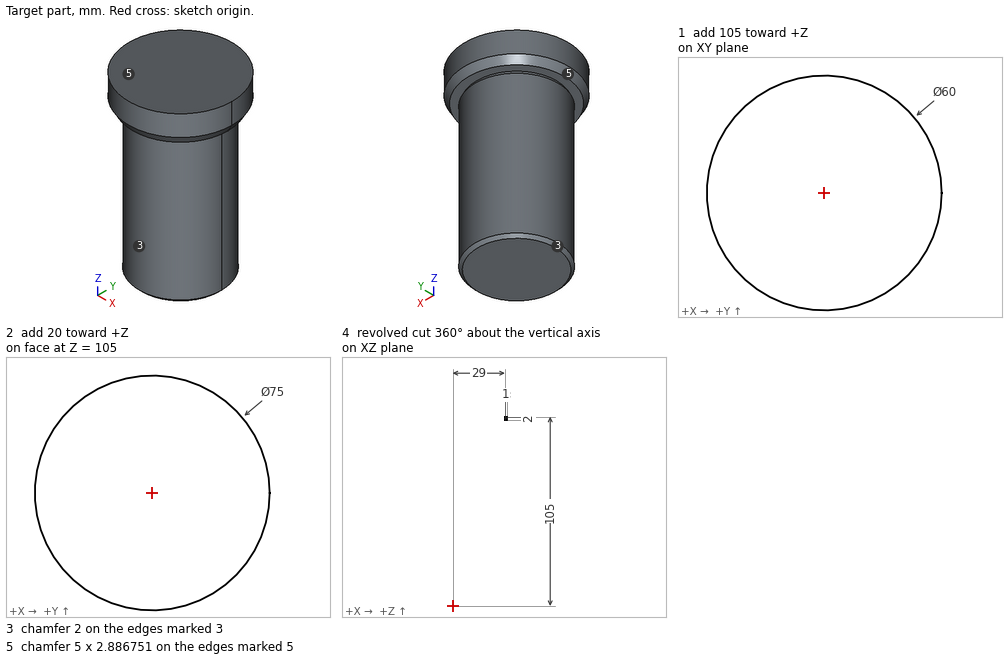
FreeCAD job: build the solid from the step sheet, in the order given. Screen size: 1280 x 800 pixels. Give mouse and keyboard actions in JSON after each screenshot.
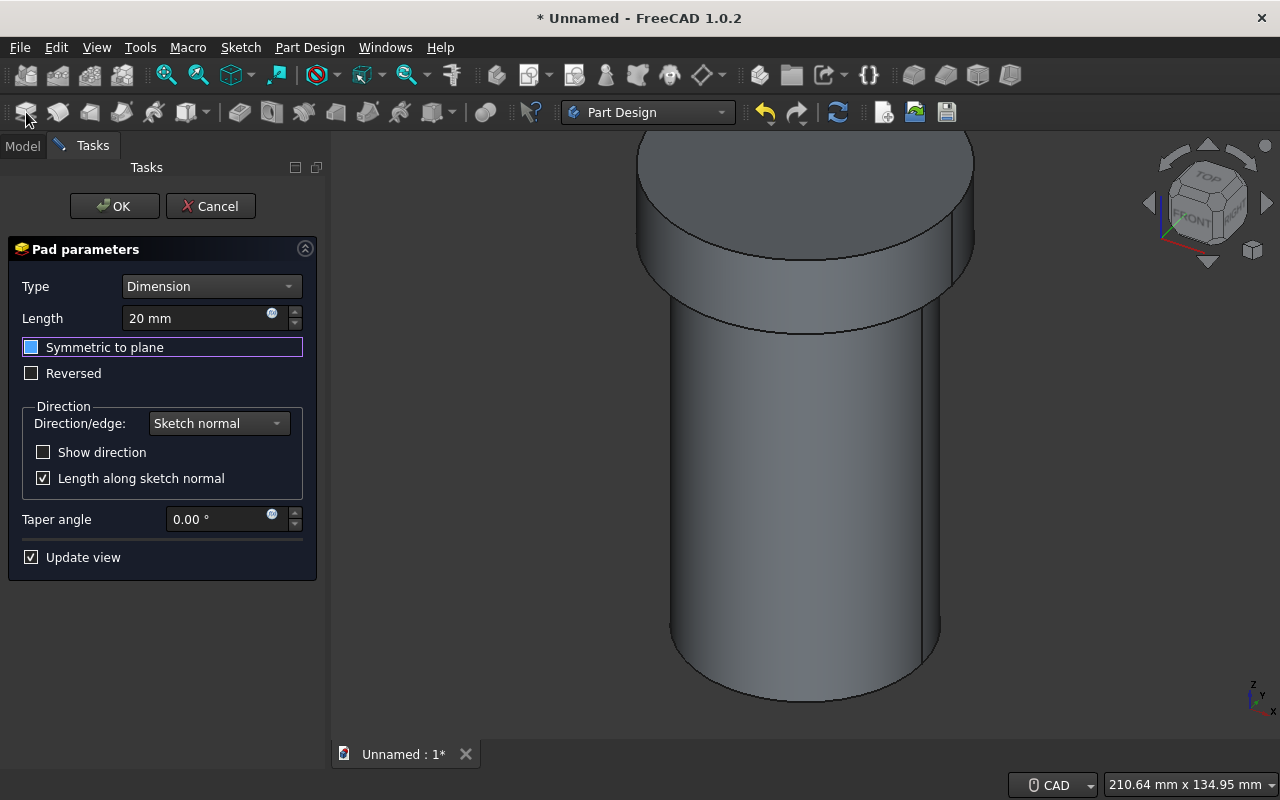
{"action": "left_click", "coordinate": [115, 206]}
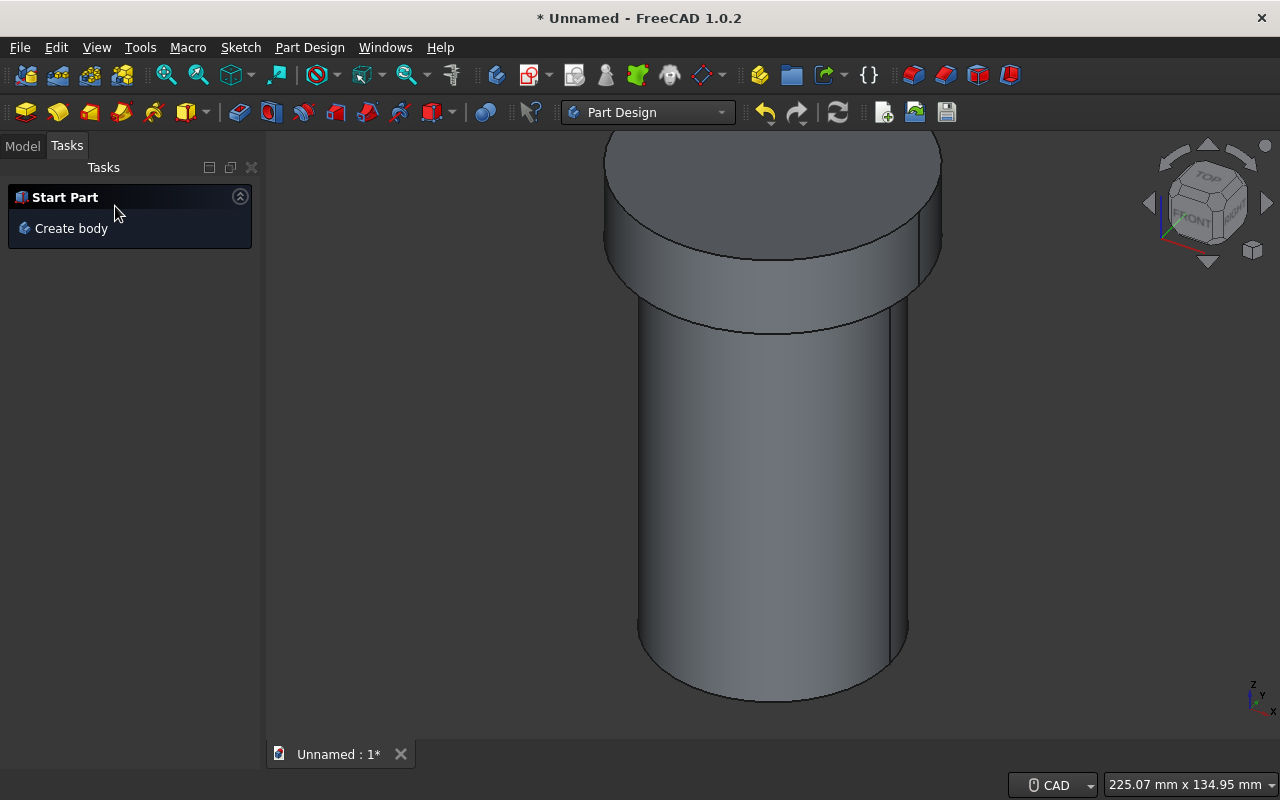
{"action": "left_click", "coordinate": [168, 76]}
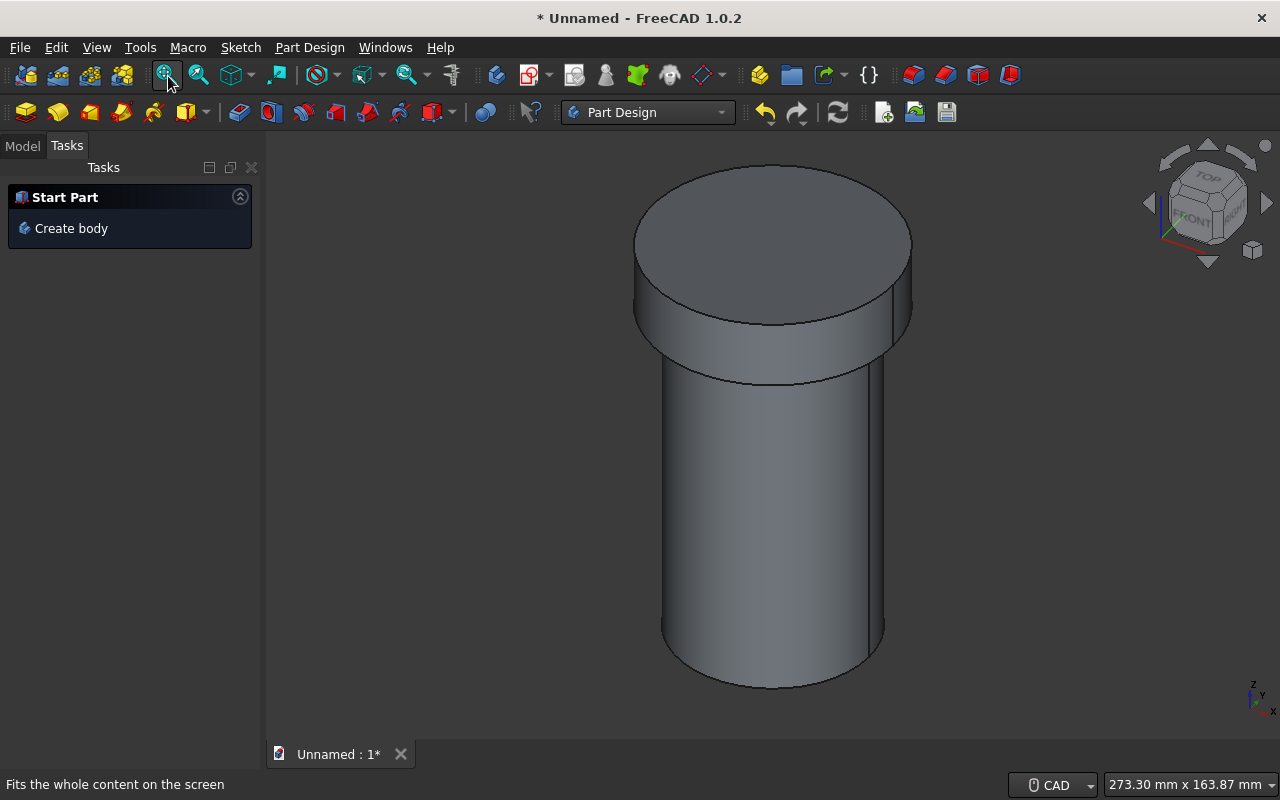
{"action": "left_click", "coordinate": [690, 667]}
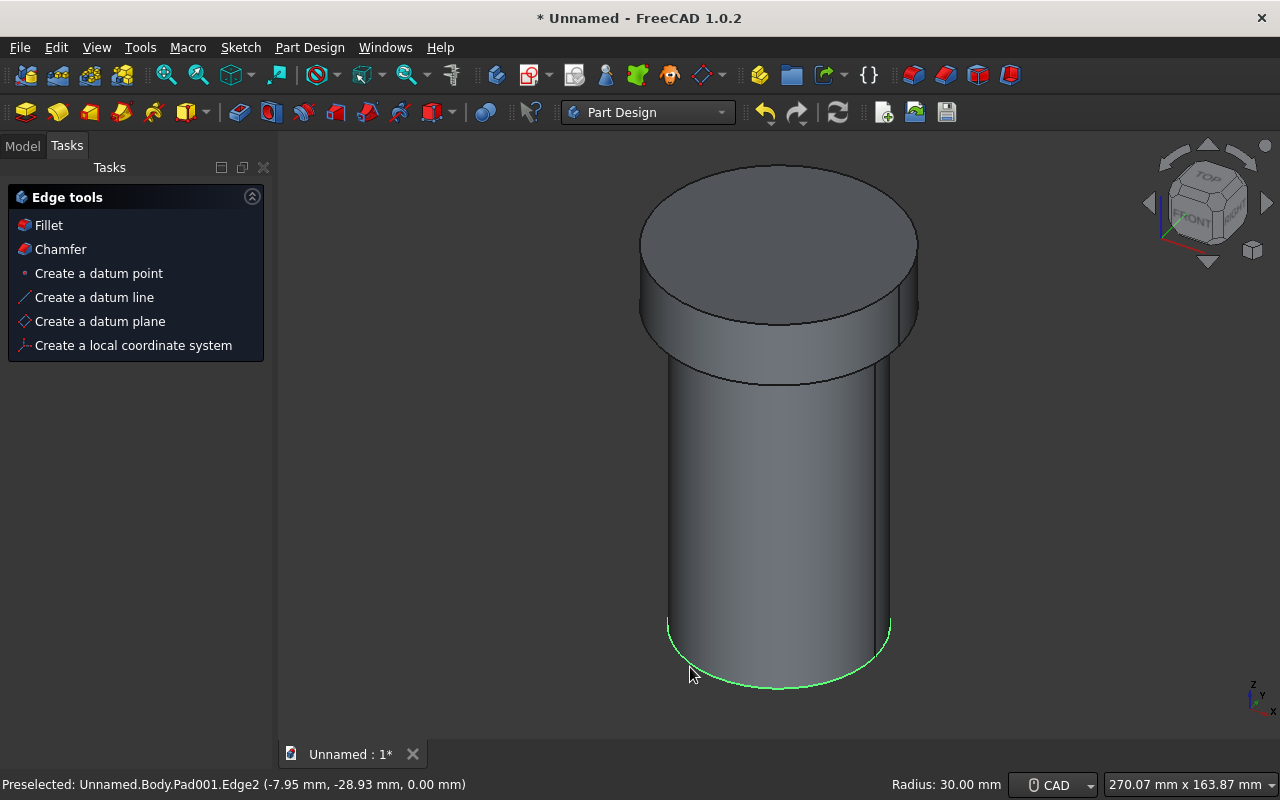
{"action": "left_click", "coordinate": [946, 76]}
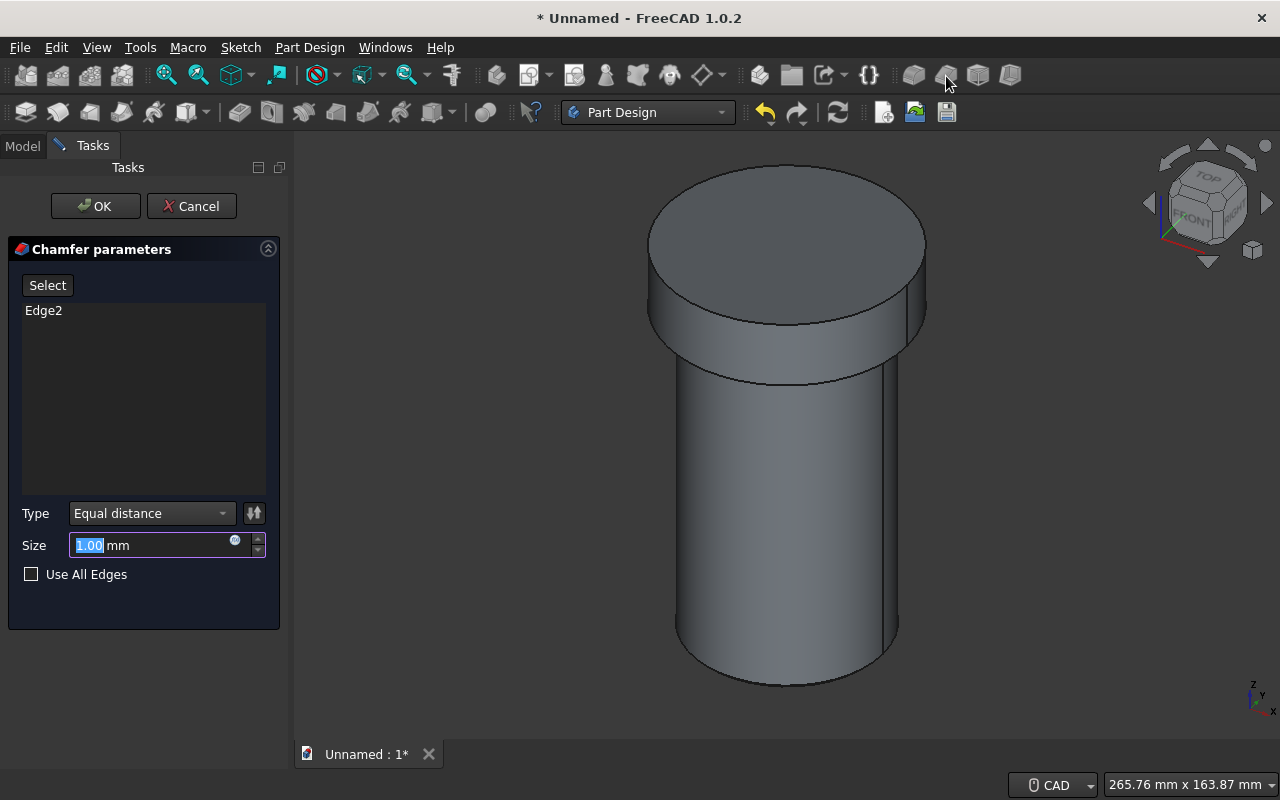
{"action": "type", "text": "2"}
{"action": "key", "text": "Tab"}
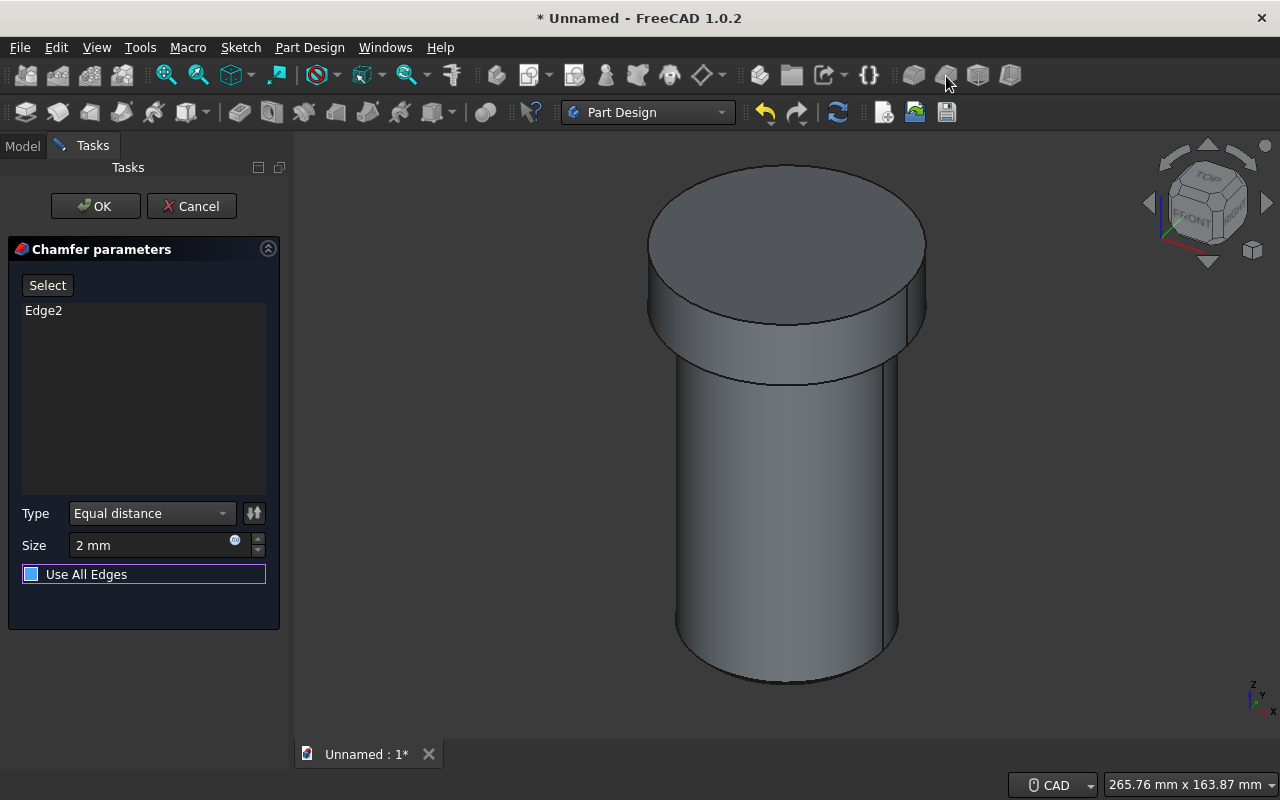
{"action": "left_click", "coordinate": [96, 206]}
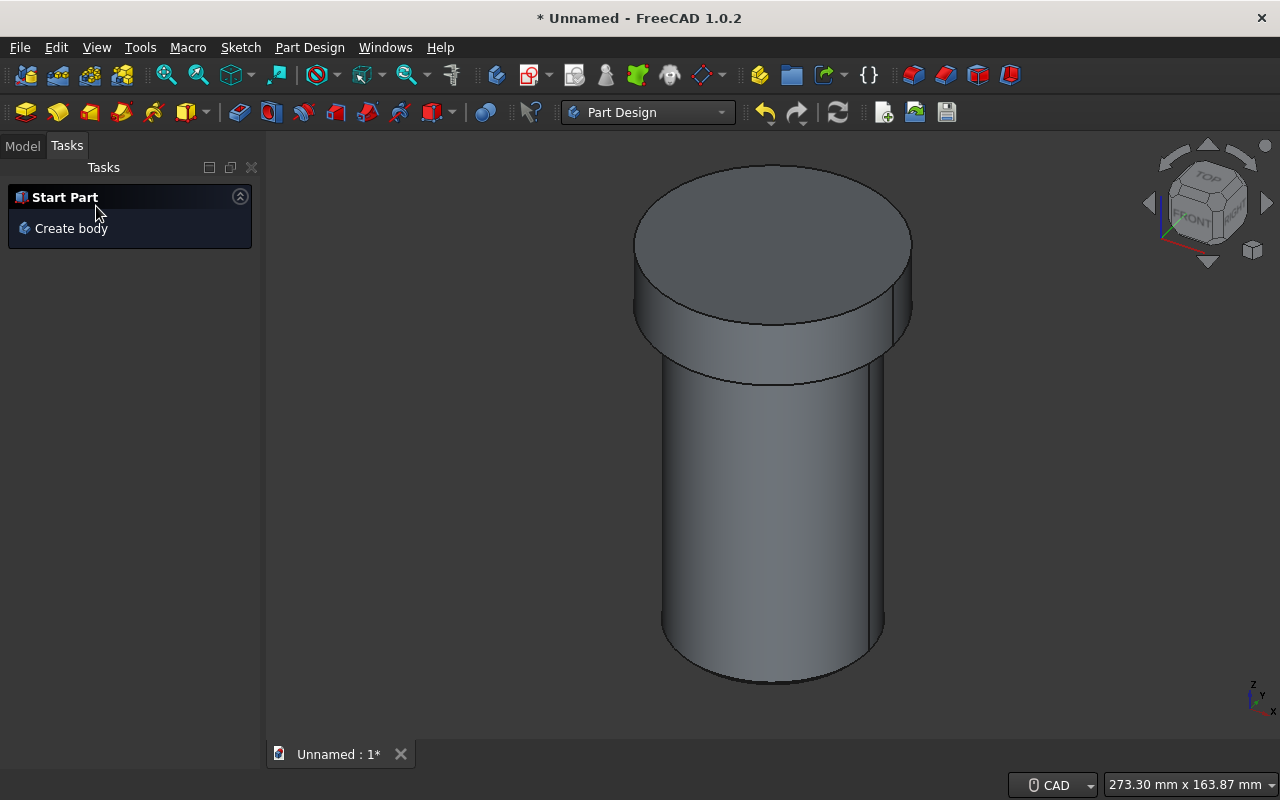
{"action": "left_click", "coordinate": [530, 76]}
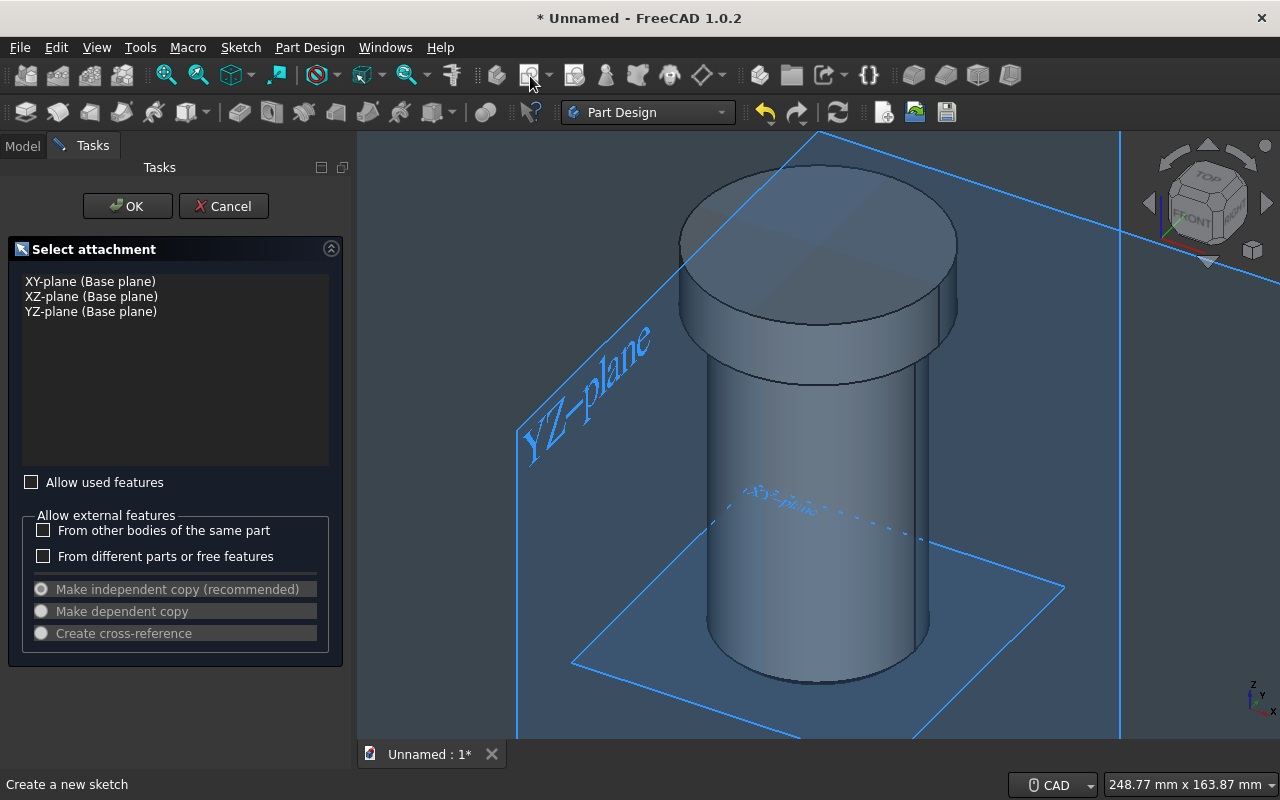
{"action": "left_click", "coordinate": [82, 296]}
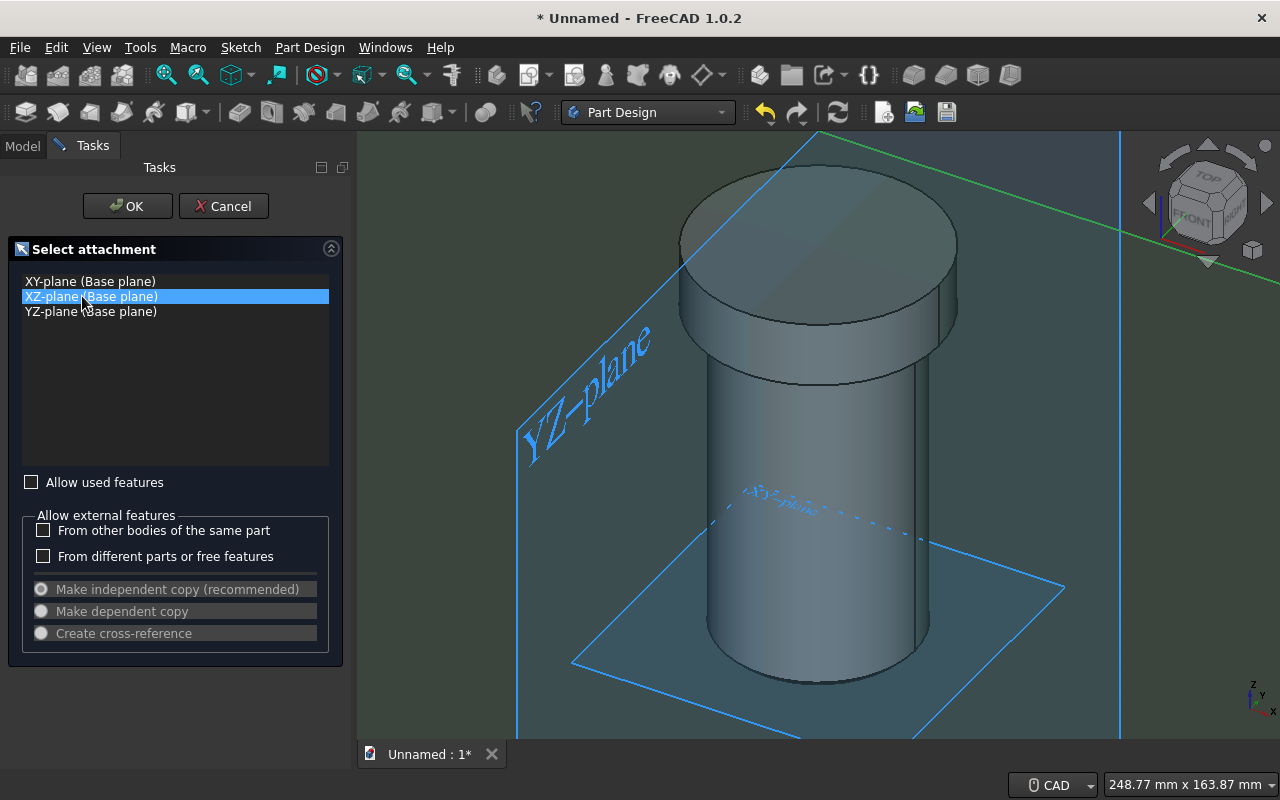
{"action": "left_click", "coordinate": [128, 206]}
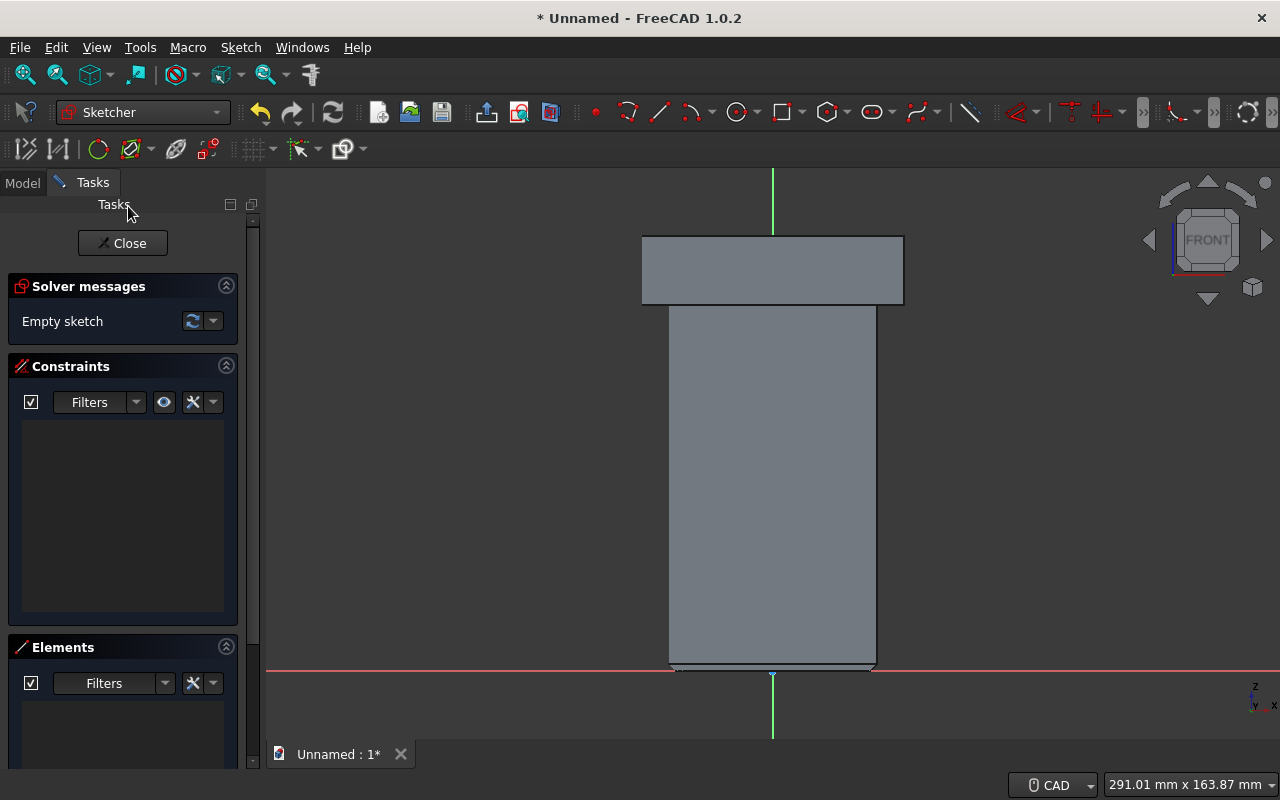
{"action": "left_click", "coordinate": [552, 112]}